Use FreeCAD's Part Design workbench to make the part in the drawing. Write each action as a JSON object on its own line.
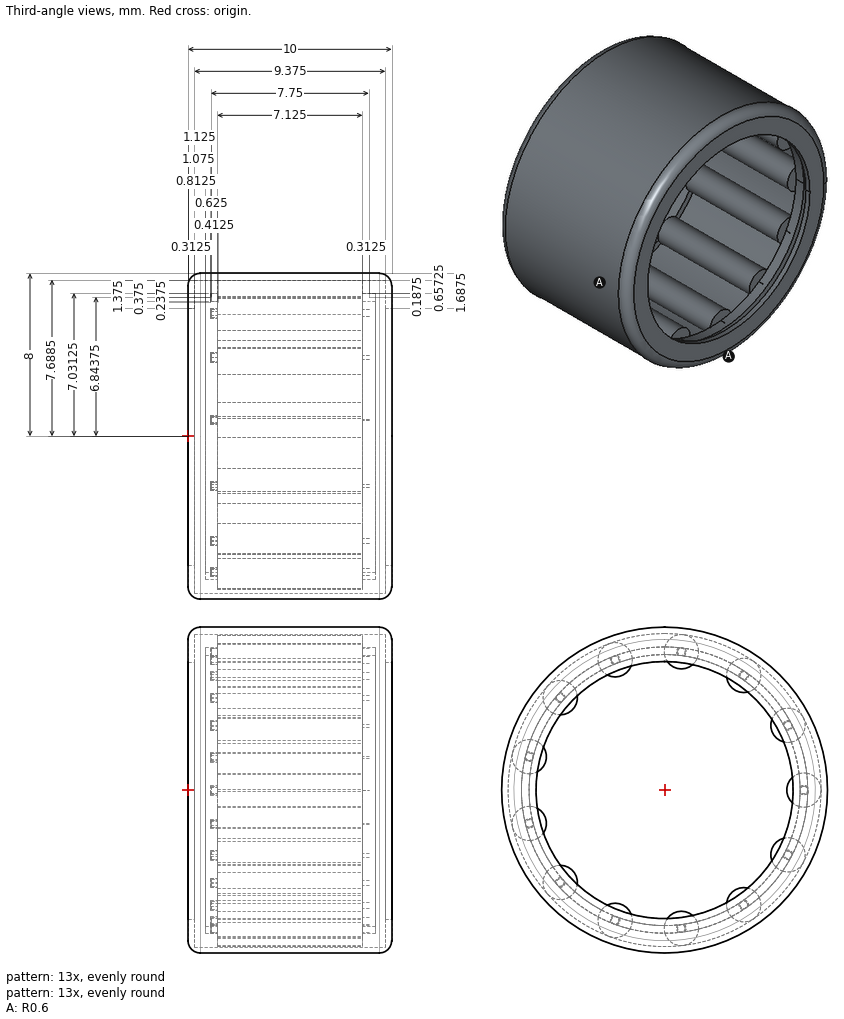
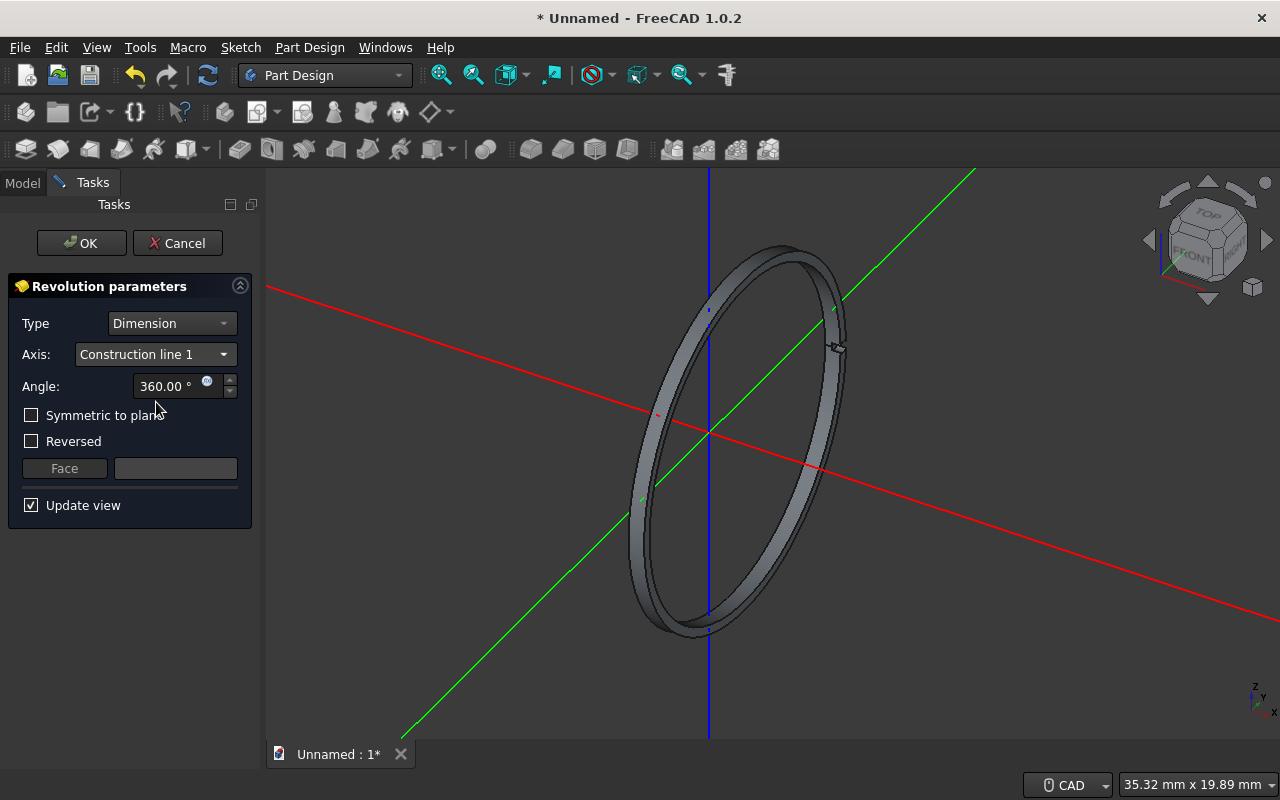
{"action": "left_click", "coordinate": [82, 243]}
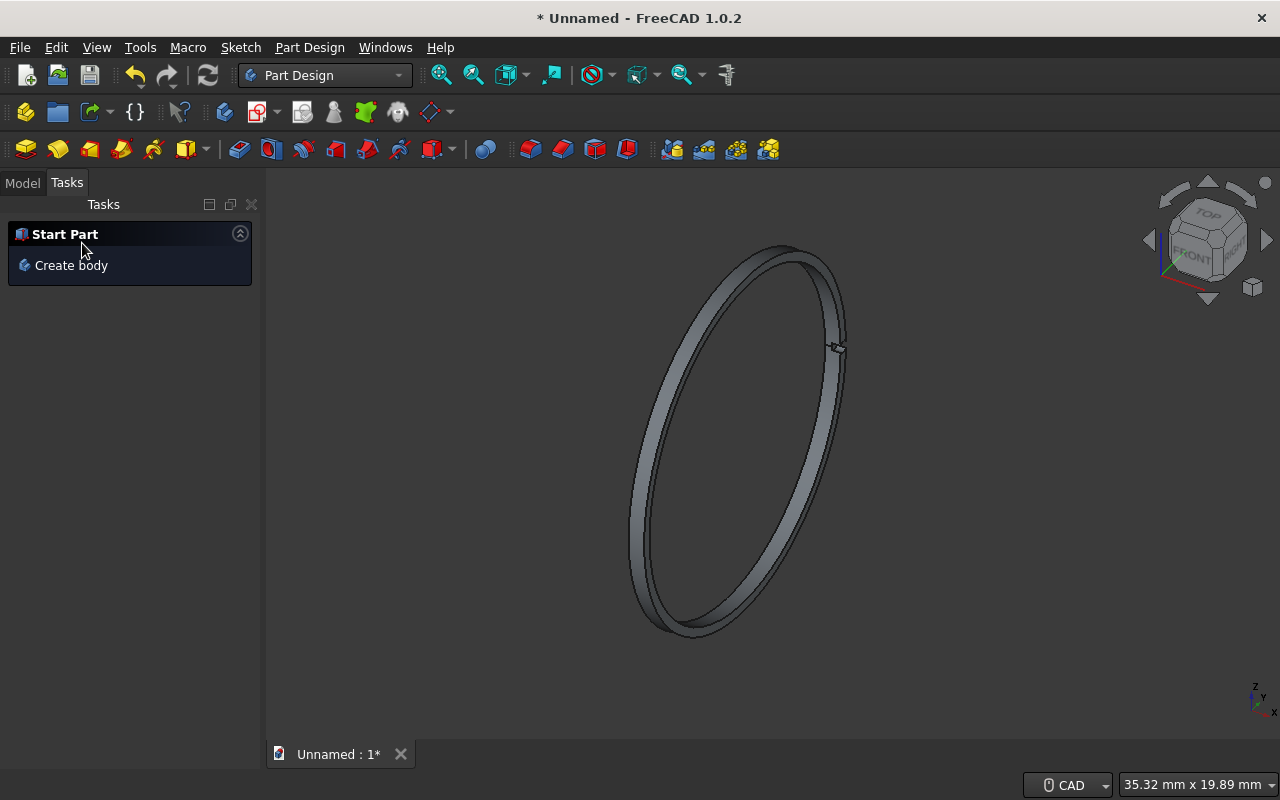
{"action": "left_click", "coordinate": [23, 182]}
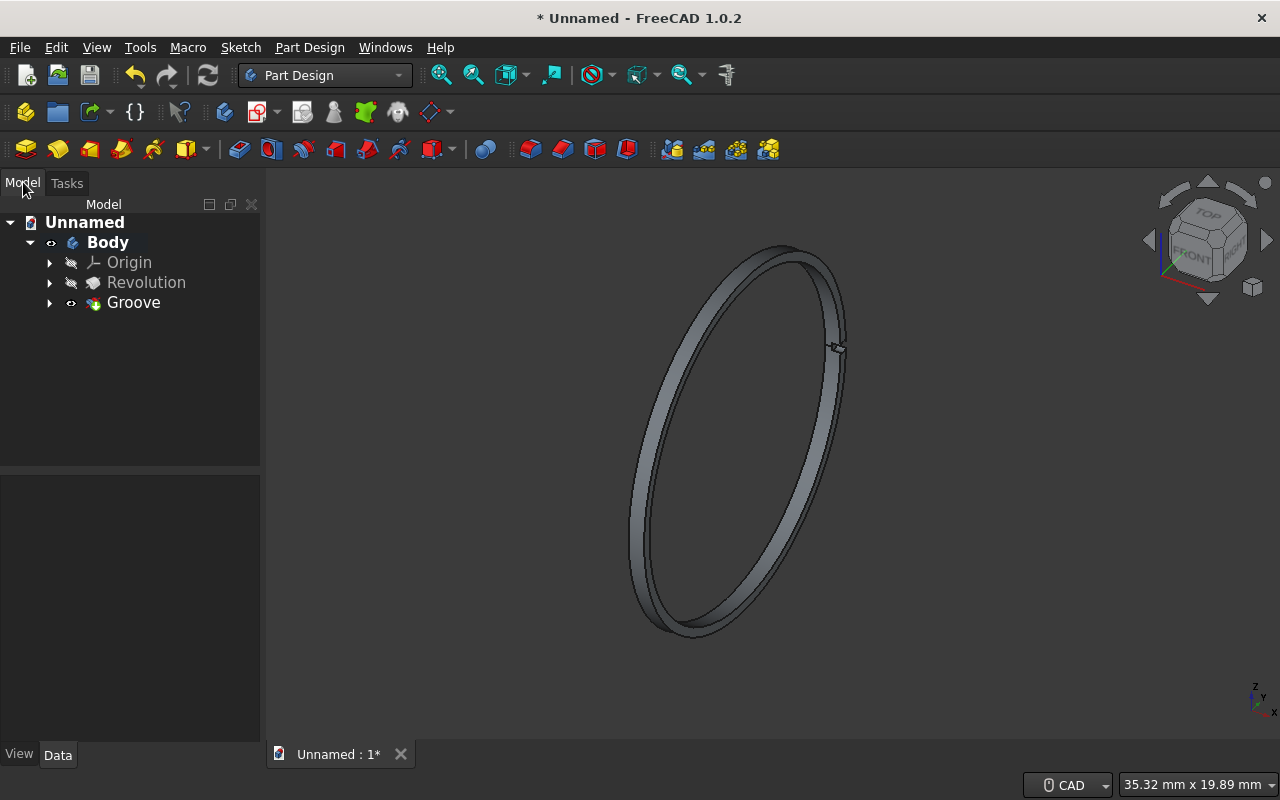
{"action": "left_click", "coordinate": [116, 303]}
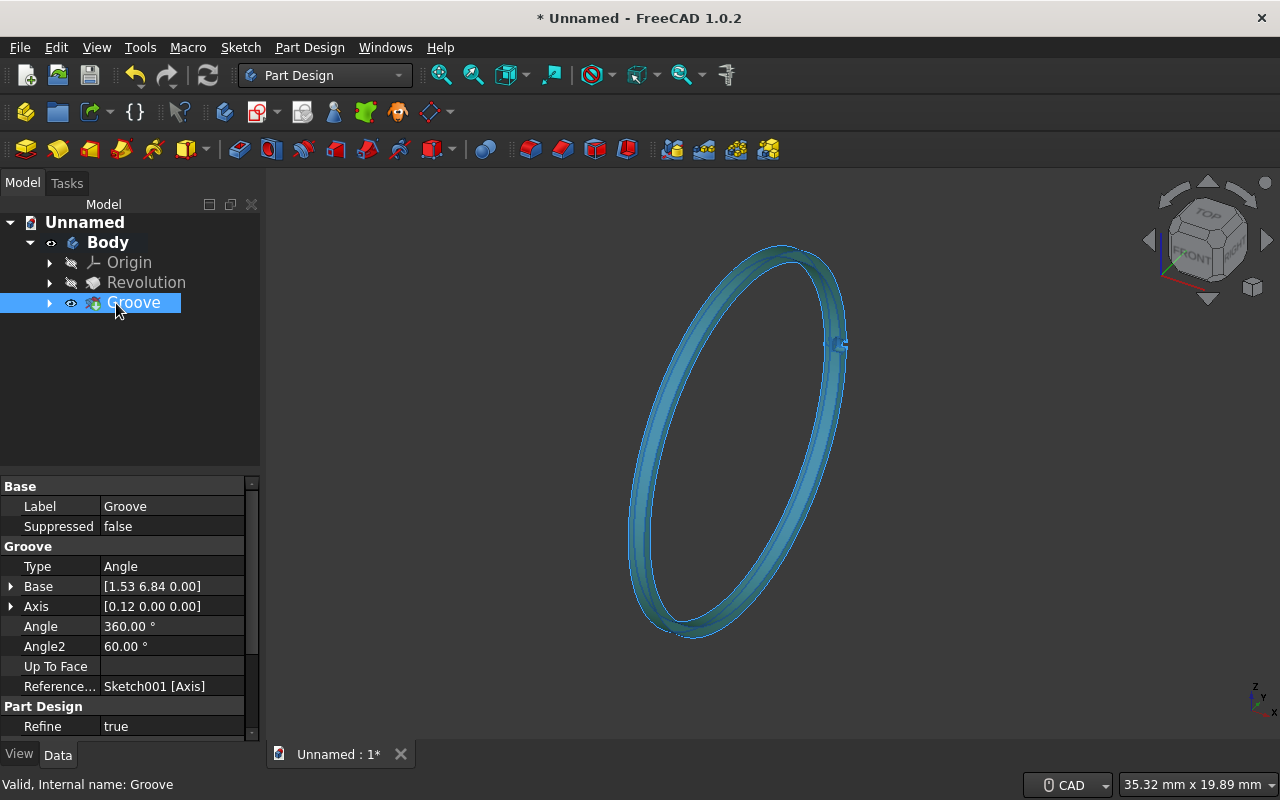
{"action": "left_click", "coordinate": [736, 150]}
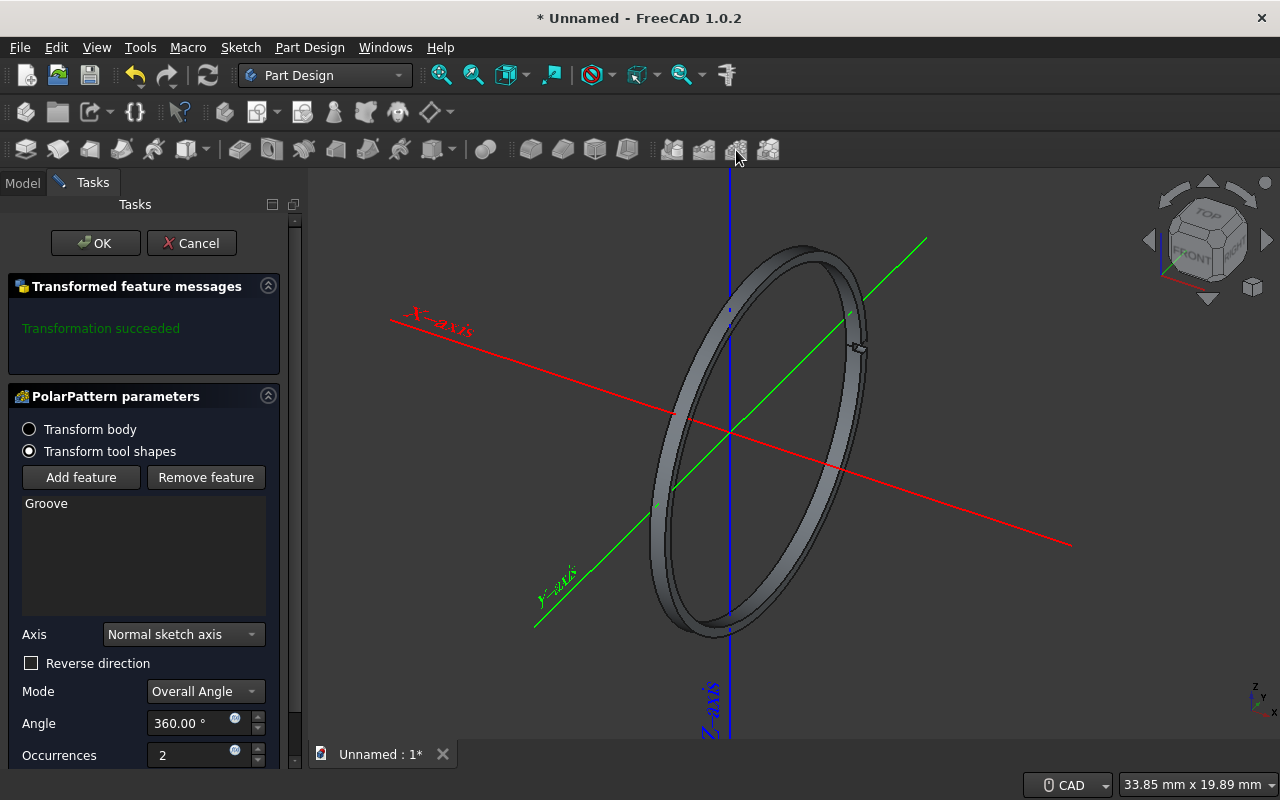
{"action": "left_click", "coordinate": [184, 634]}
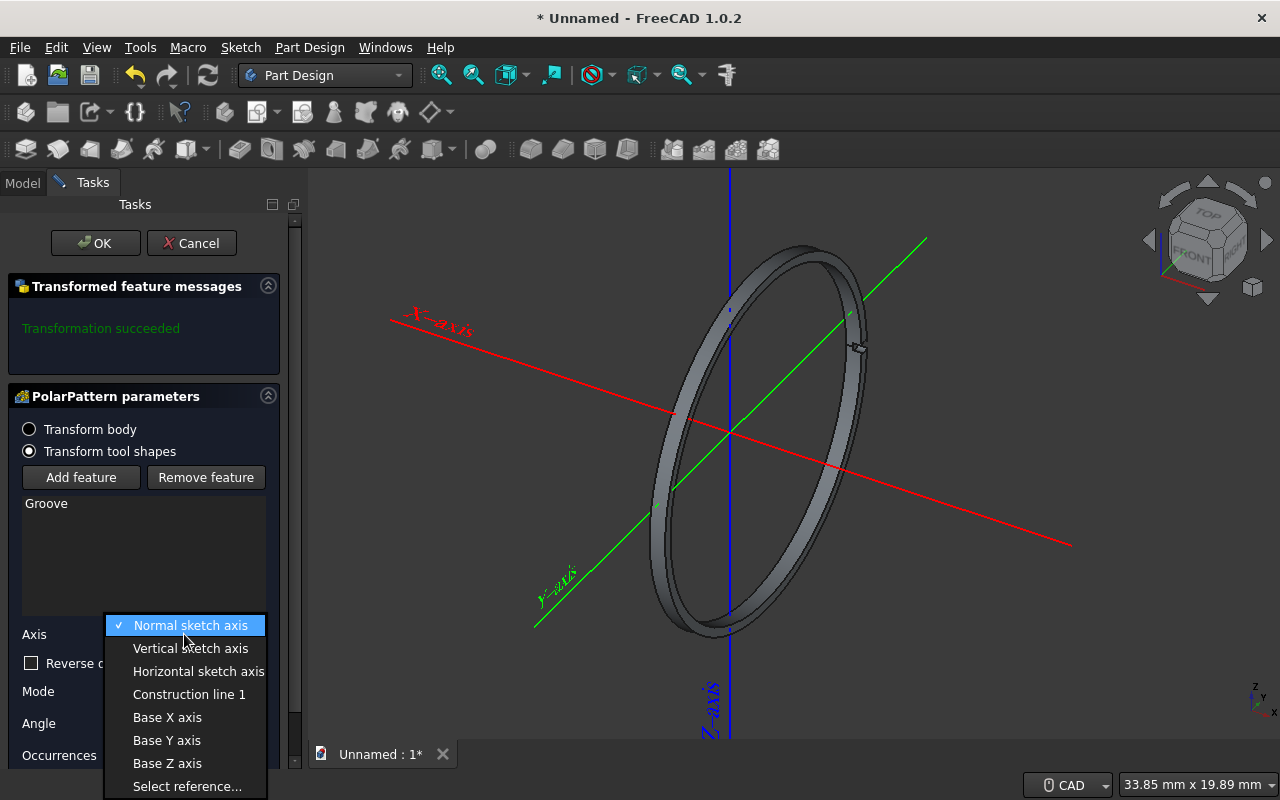
{"action": "left_click", "coordinate": [184, 718]}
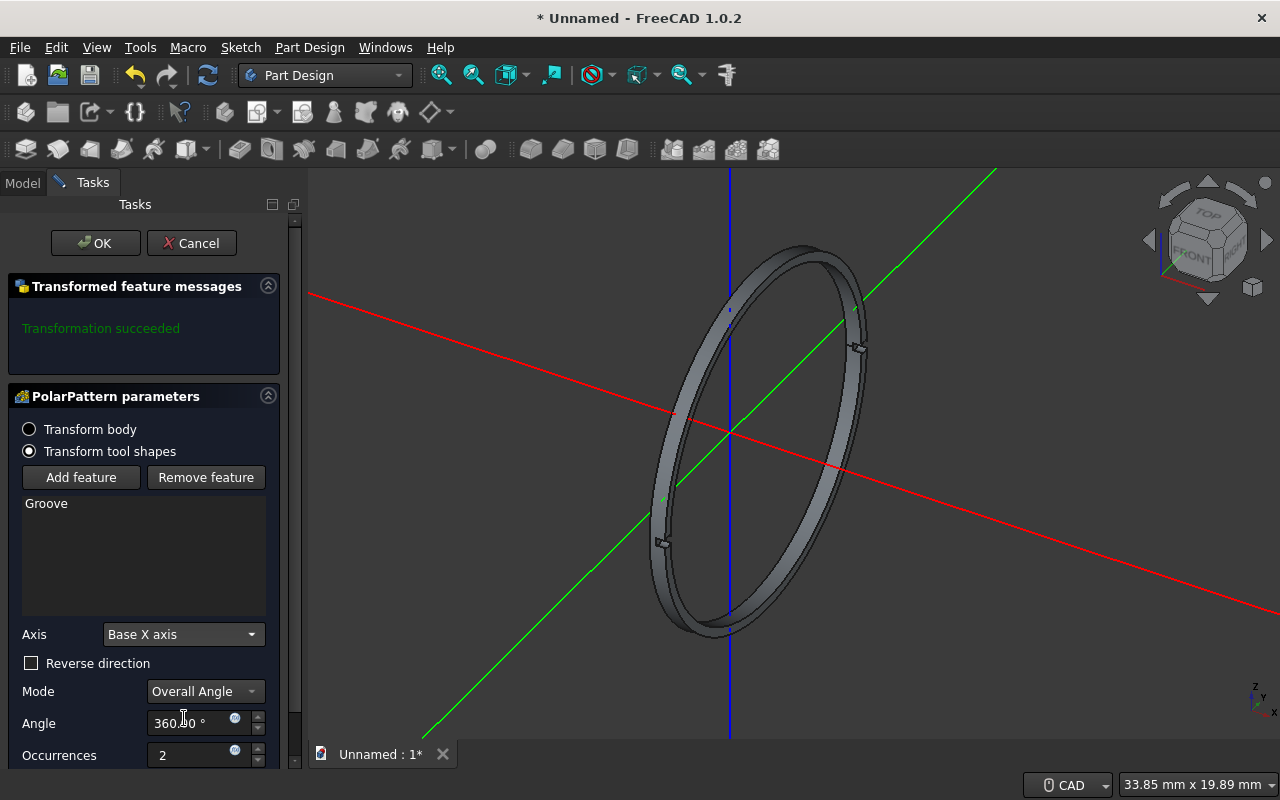
{"action": "triple_click", "coordinate": [198, 755]}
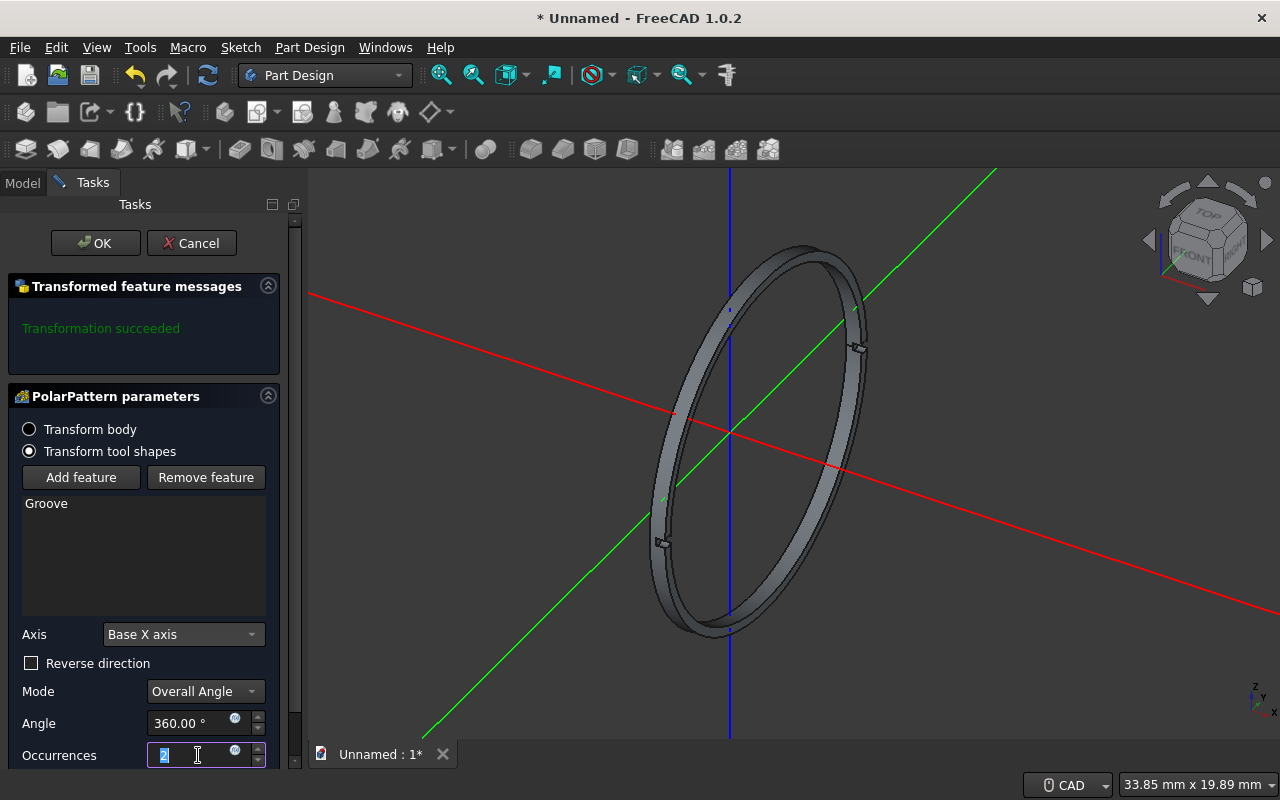
{"action": "type", "text": "13"}
{"action": "key", "text": "Tab"}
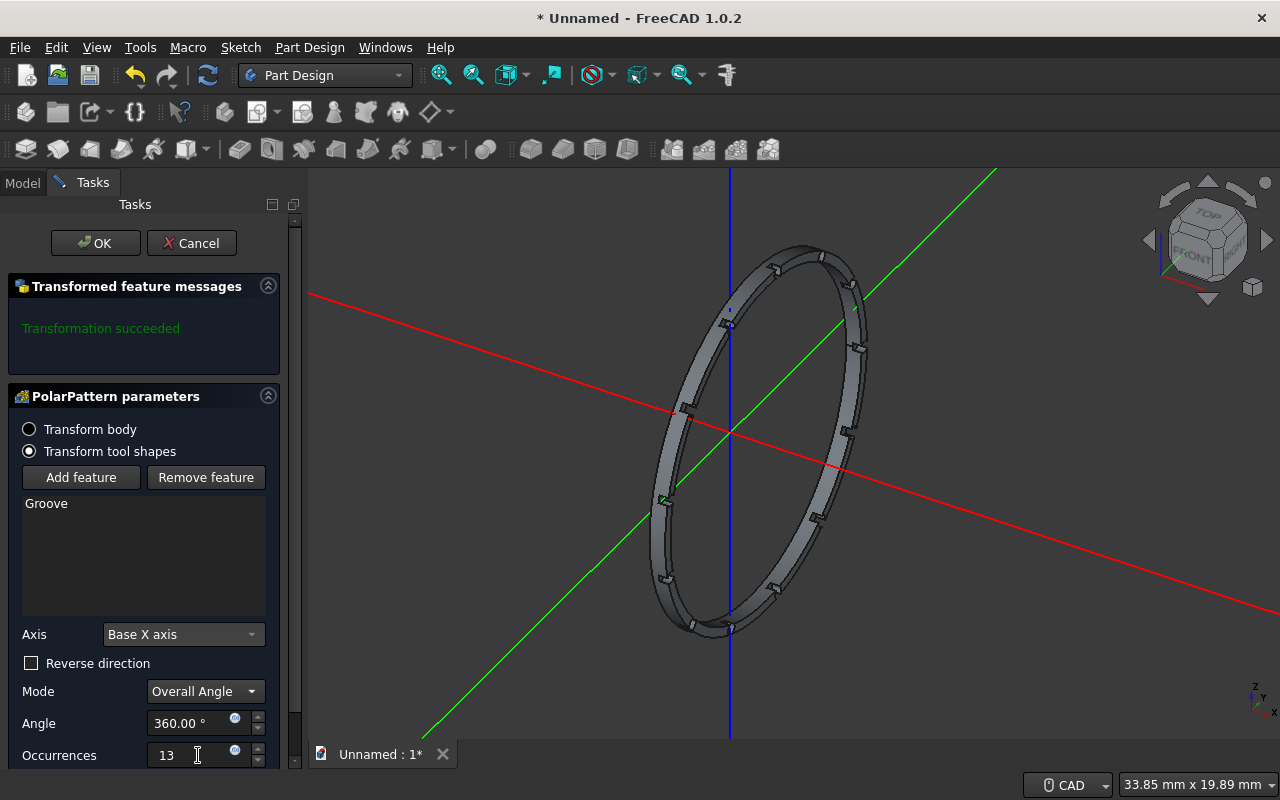
{"action": "left_click", "coordinate": [96, 243]}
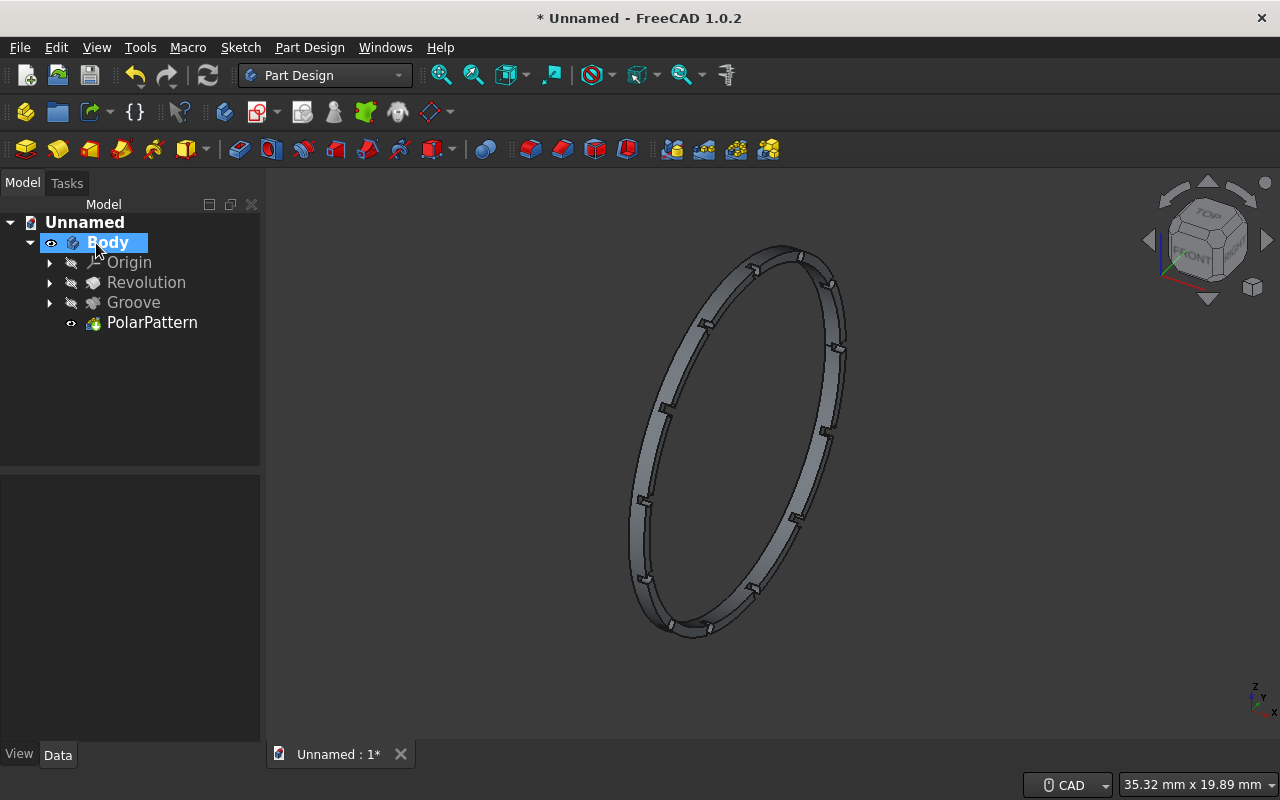
{"action": "left_click", "coordinate": [258, 112]}